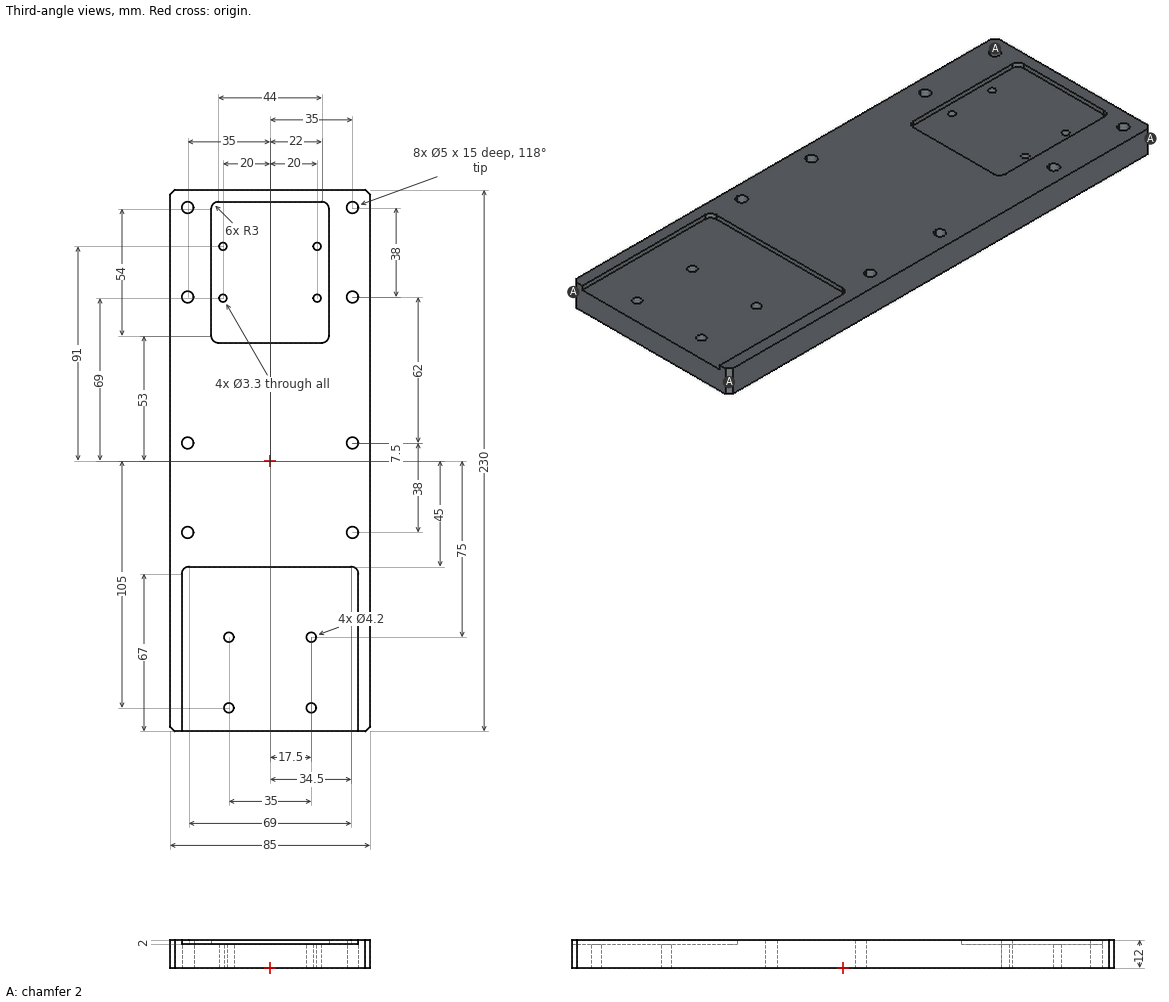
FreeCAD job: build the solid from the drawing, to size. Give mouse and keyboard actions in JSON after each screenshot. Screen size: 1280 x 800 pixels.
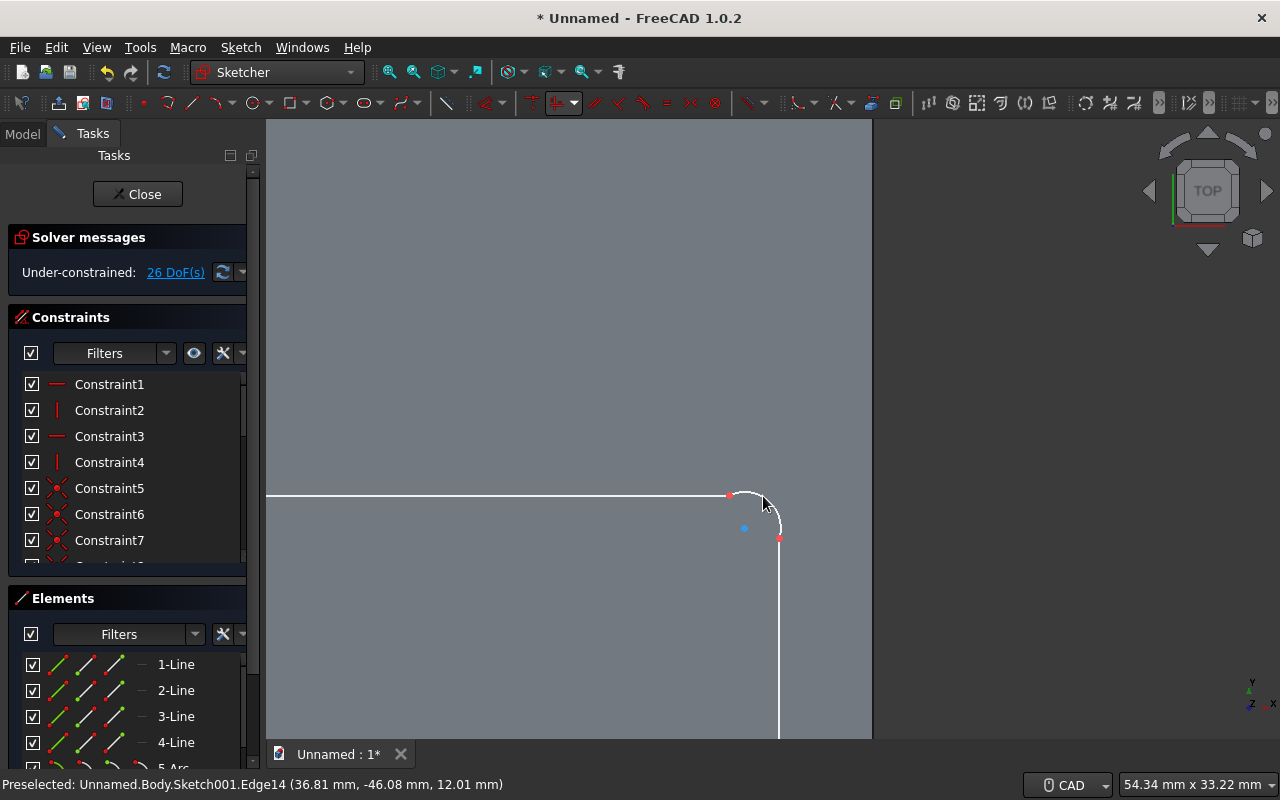
{"action": "scroll", "coordinate": [767, 503], "scroll_direction": "down", "scroll_amount": 12}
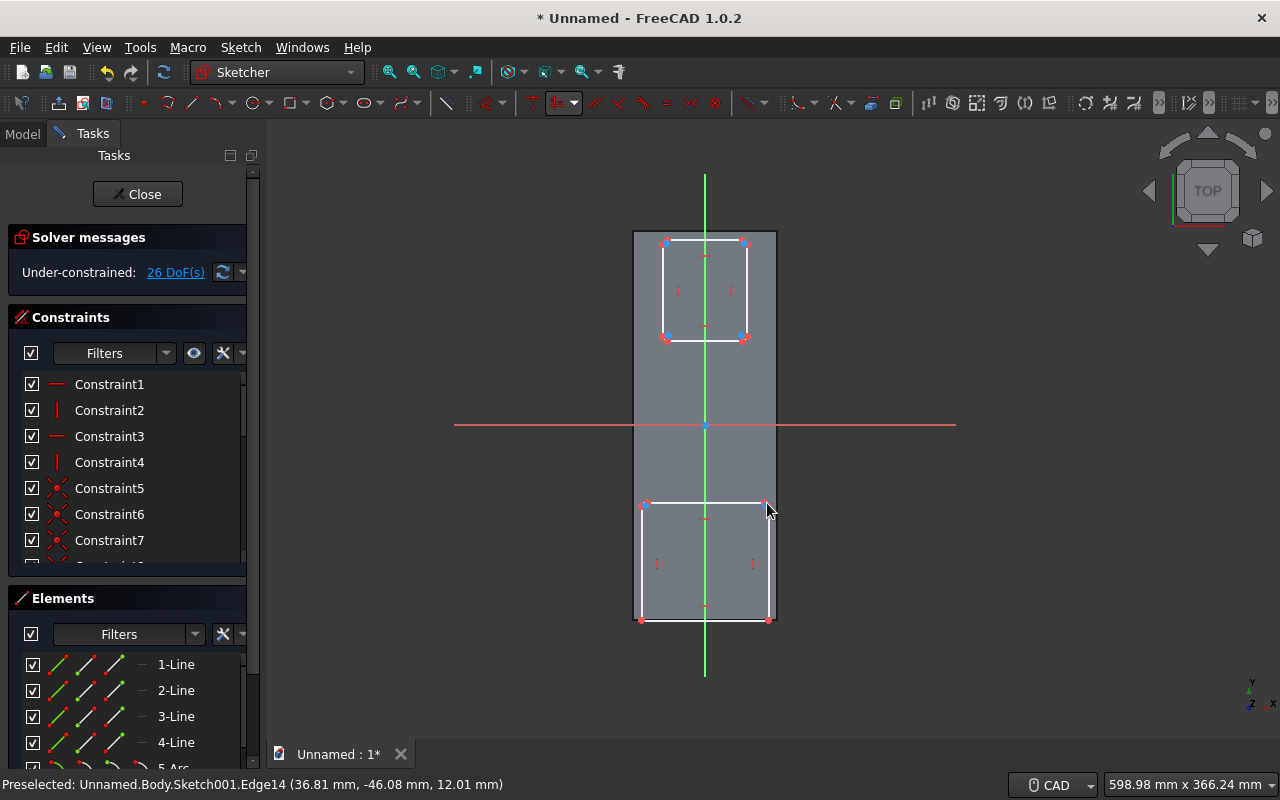
{"action": "left_click", "coordinate": [720, 240]}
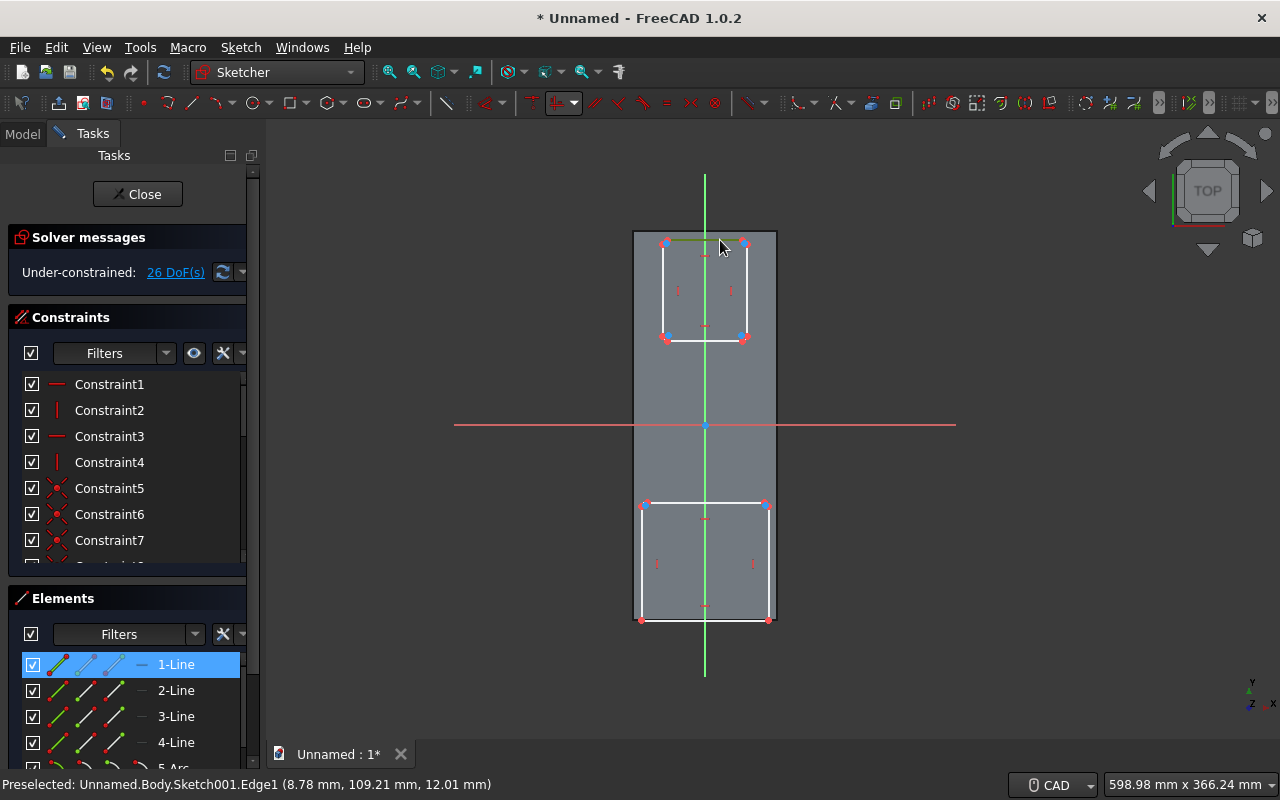
{"action": "scroll", "coordinate": [664, 241], "scroll_direction": "up", "scroll_amount": 7}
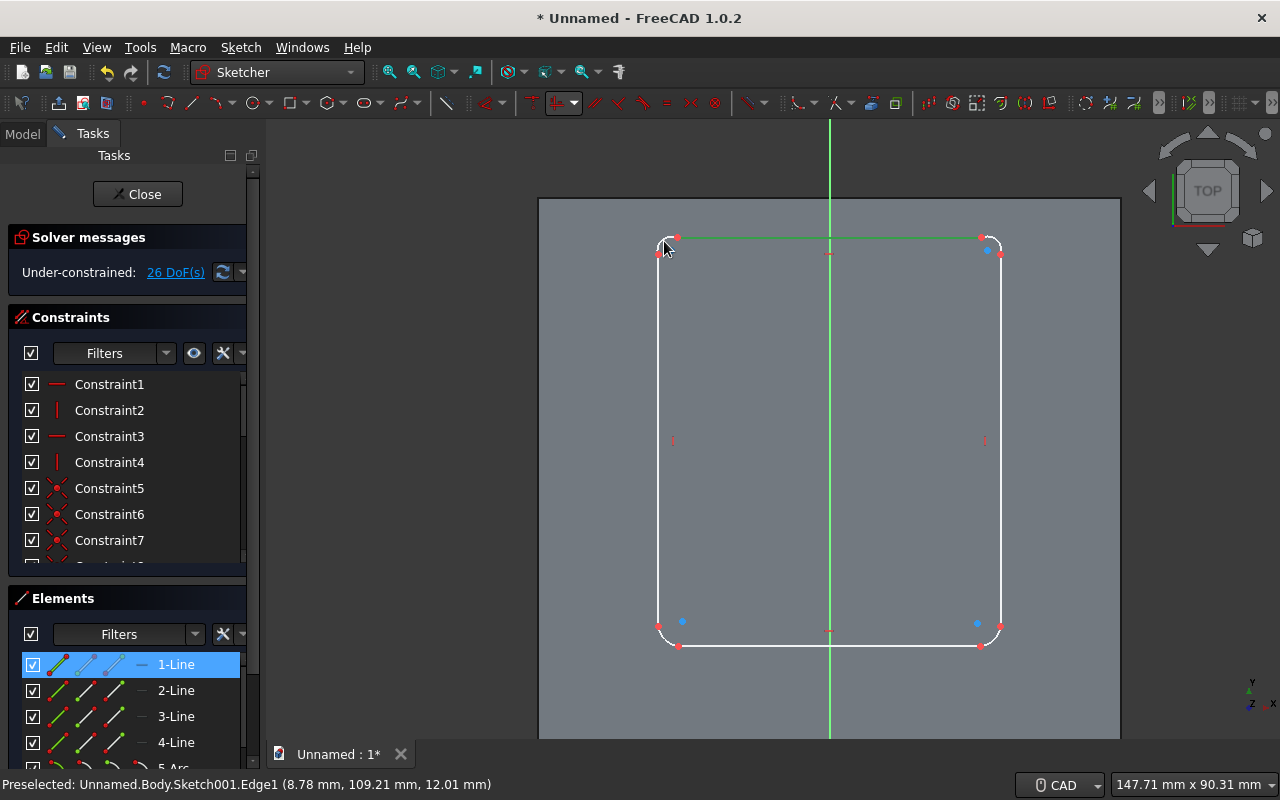
{"action": "left_click", "coordinate": [662, 240]}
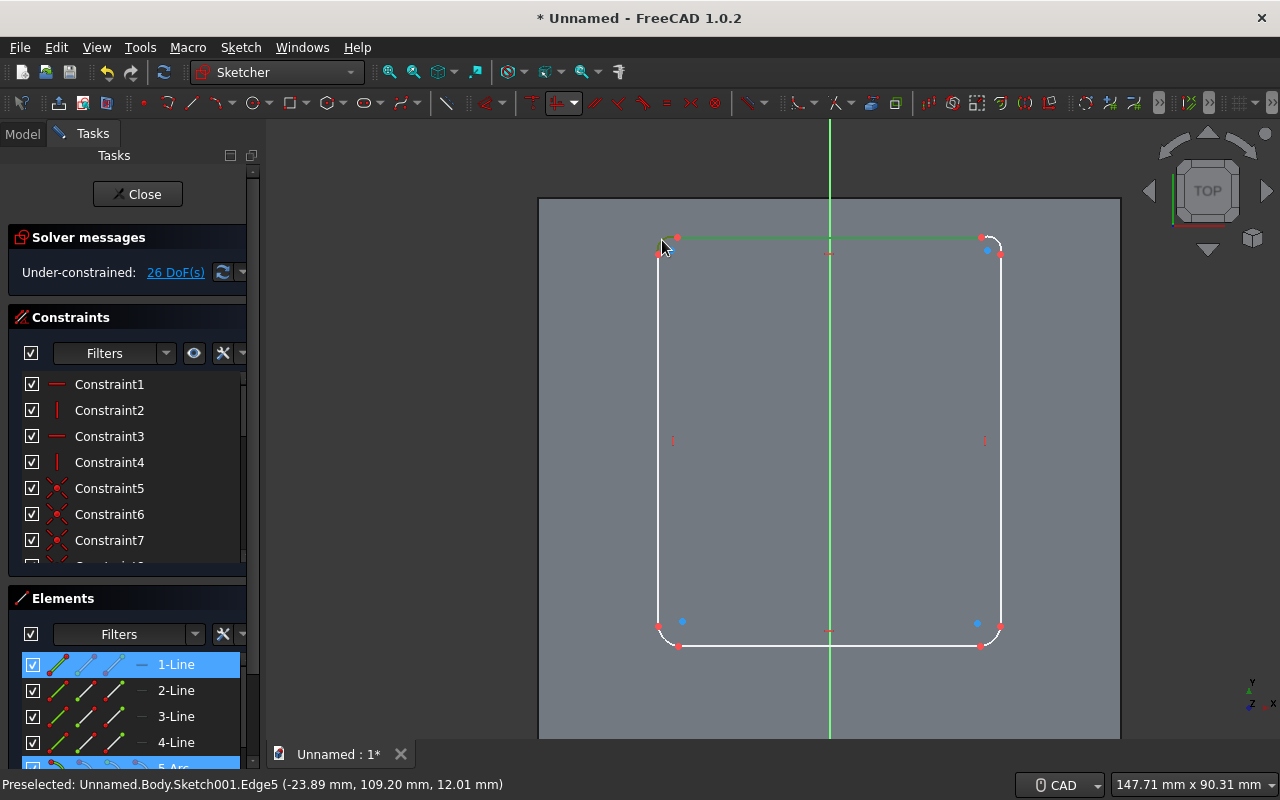
{"action": "left_click", "coordinate": [644, 104]}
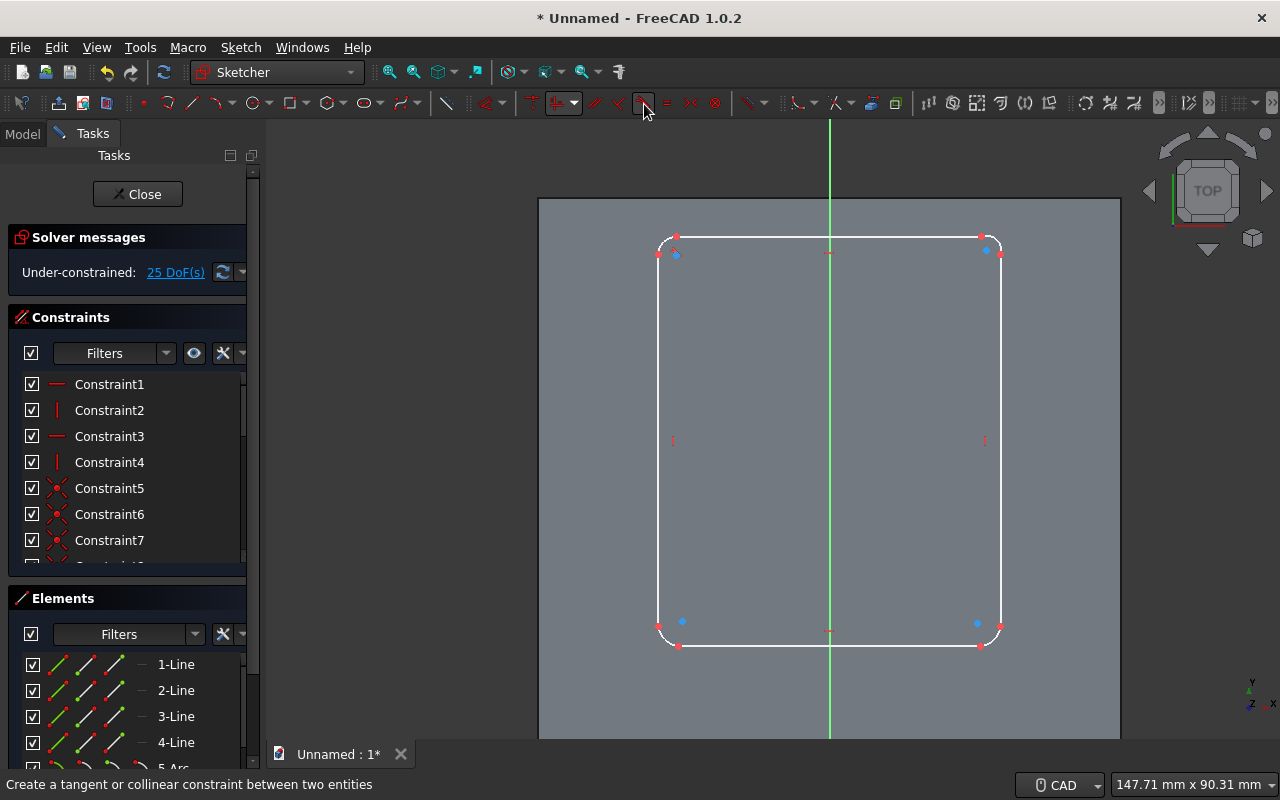
{"action": "scroll", "coordinate": [664, 241], "scroll_direction": "down", "scroll_amount": 7}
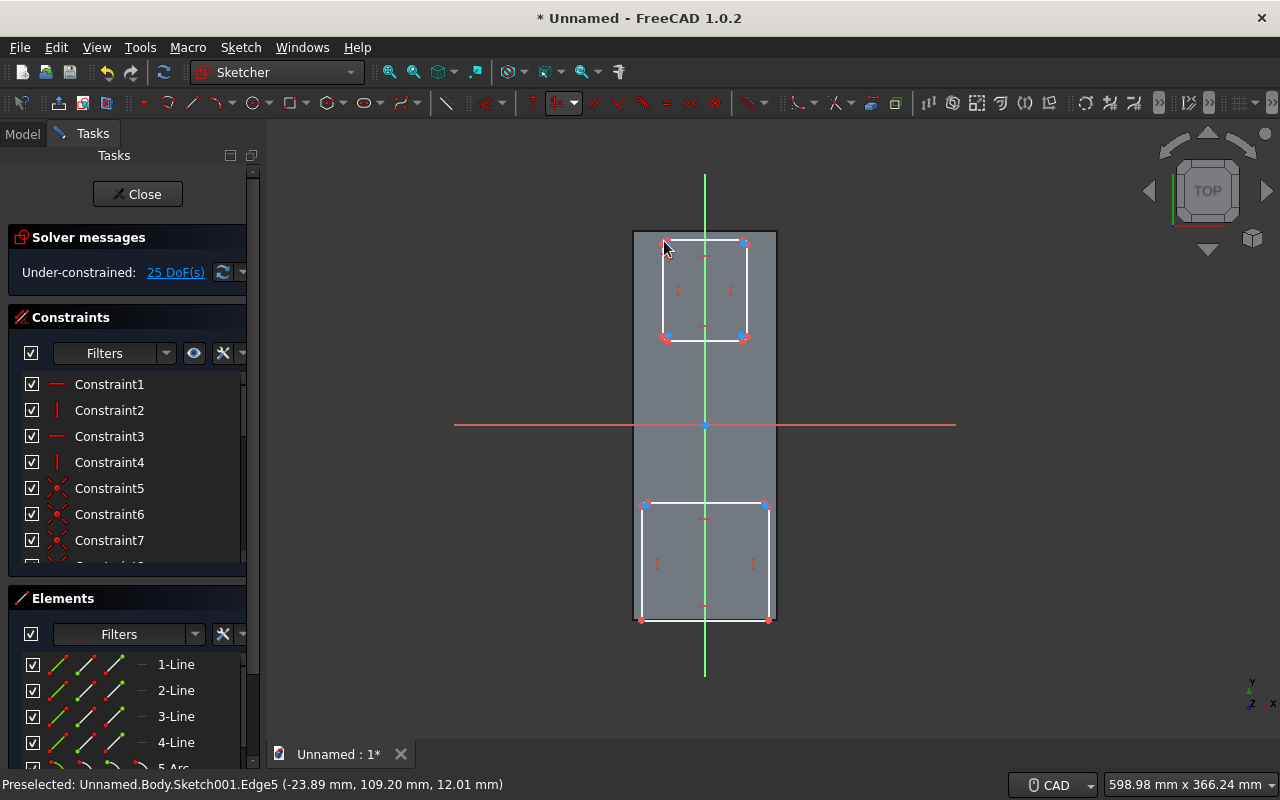
{"action": "left_click", "coordinate": [720, 240]}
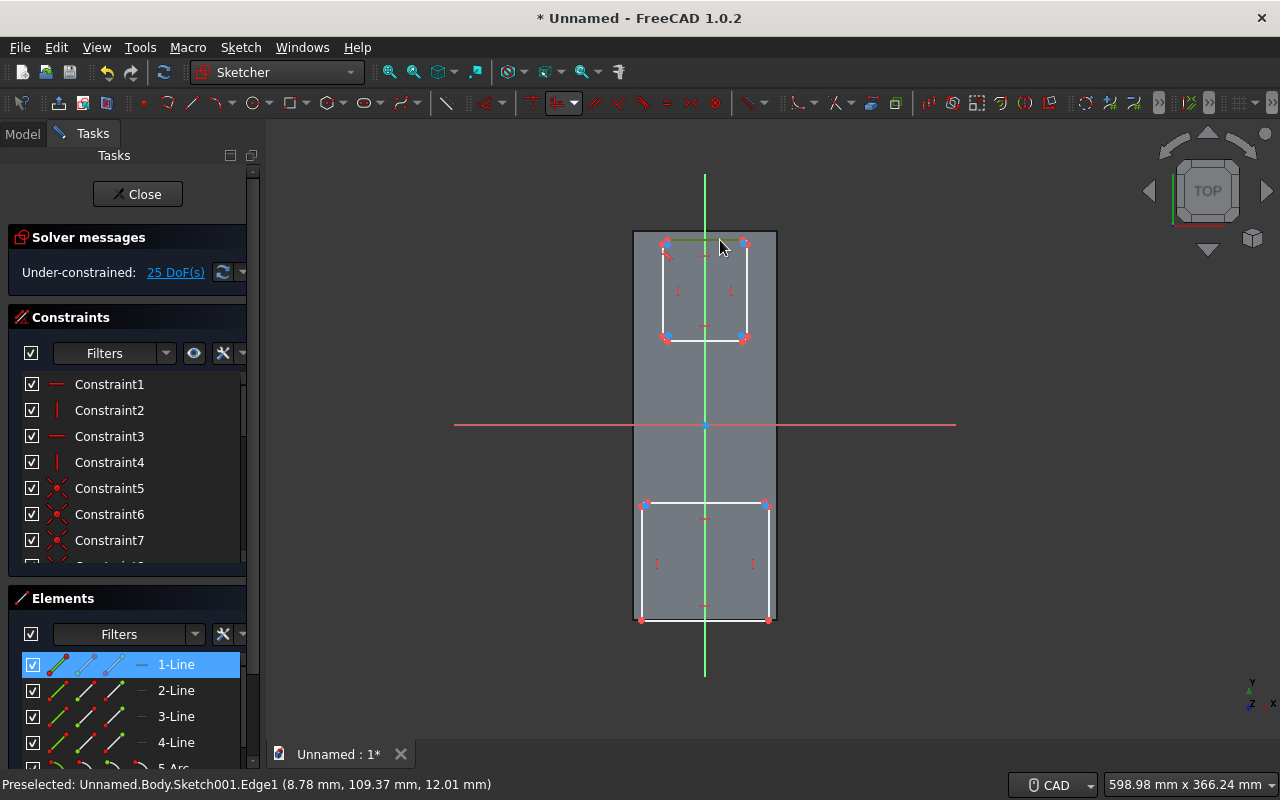
{"action": "scroll", "coordinate": [746, 241], "scroll_direction": "up", "scroll_amount": 7}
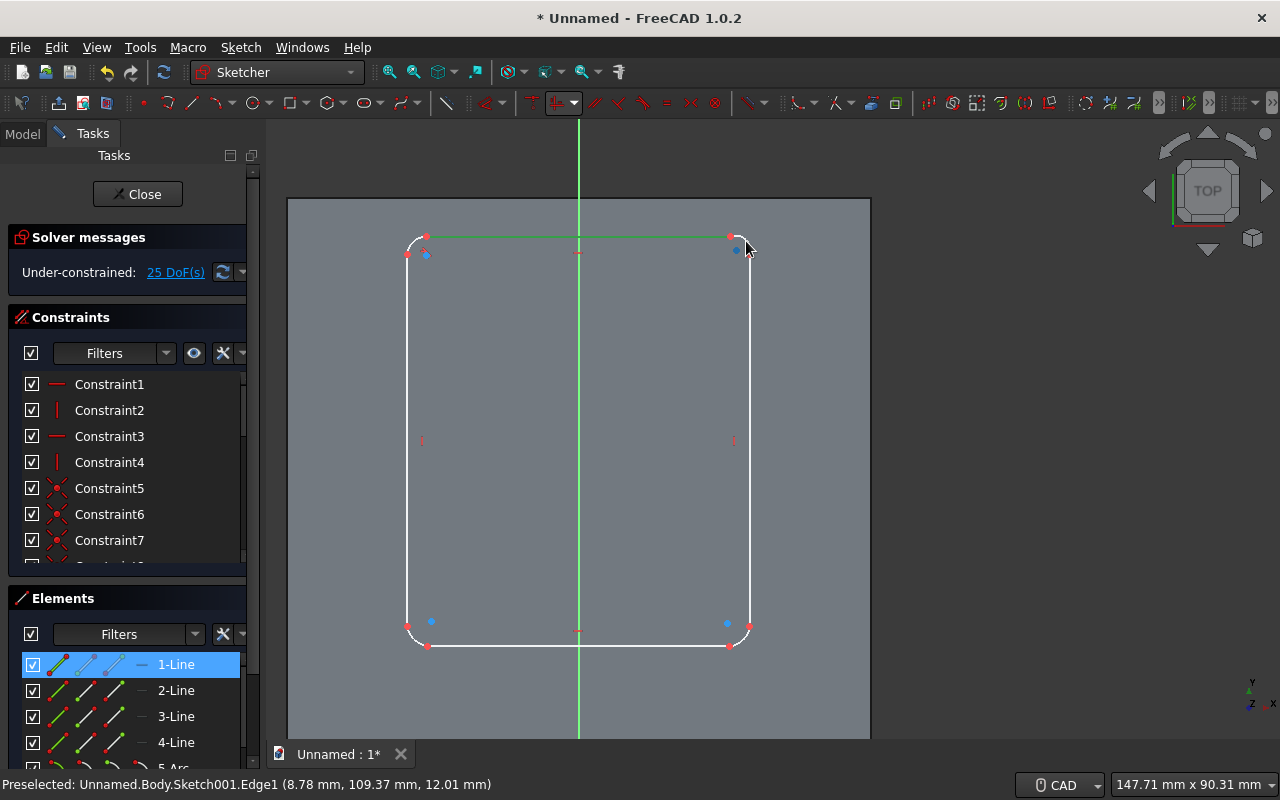
{"action": "left_click", "coordinate": [746, 240]}